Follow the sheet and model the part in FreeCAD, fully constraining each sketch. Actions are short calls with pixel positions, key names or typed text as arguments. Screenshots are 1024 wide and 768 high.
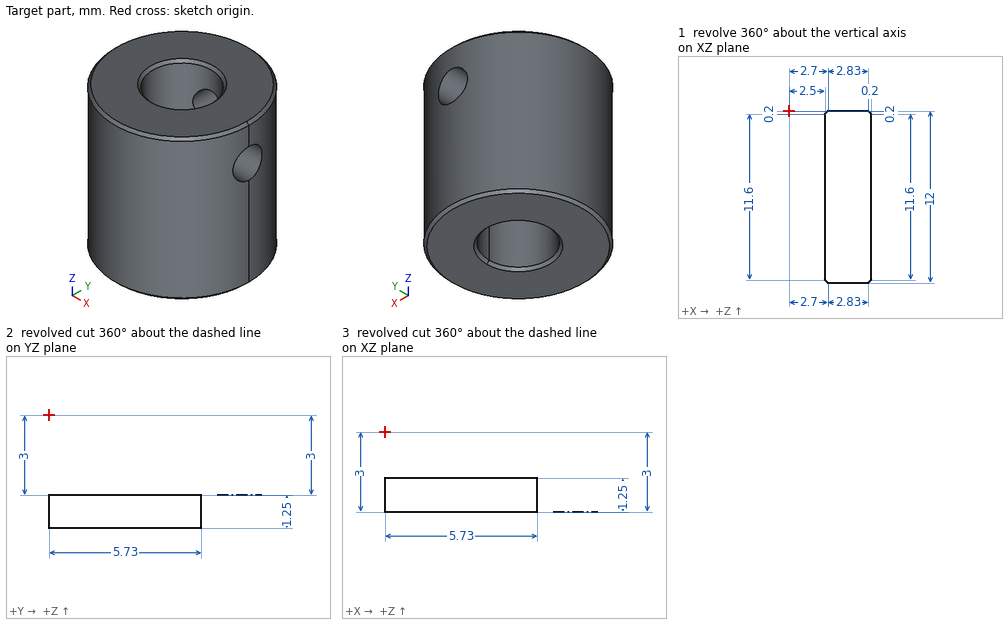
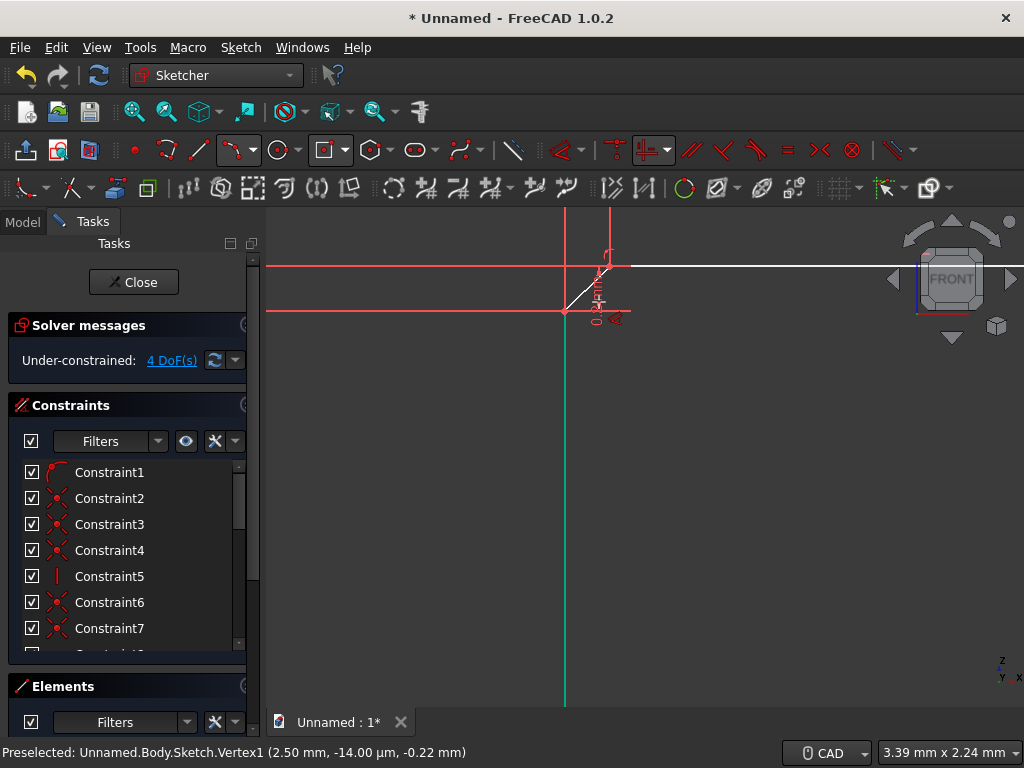
scroll(568, 314, down, 11)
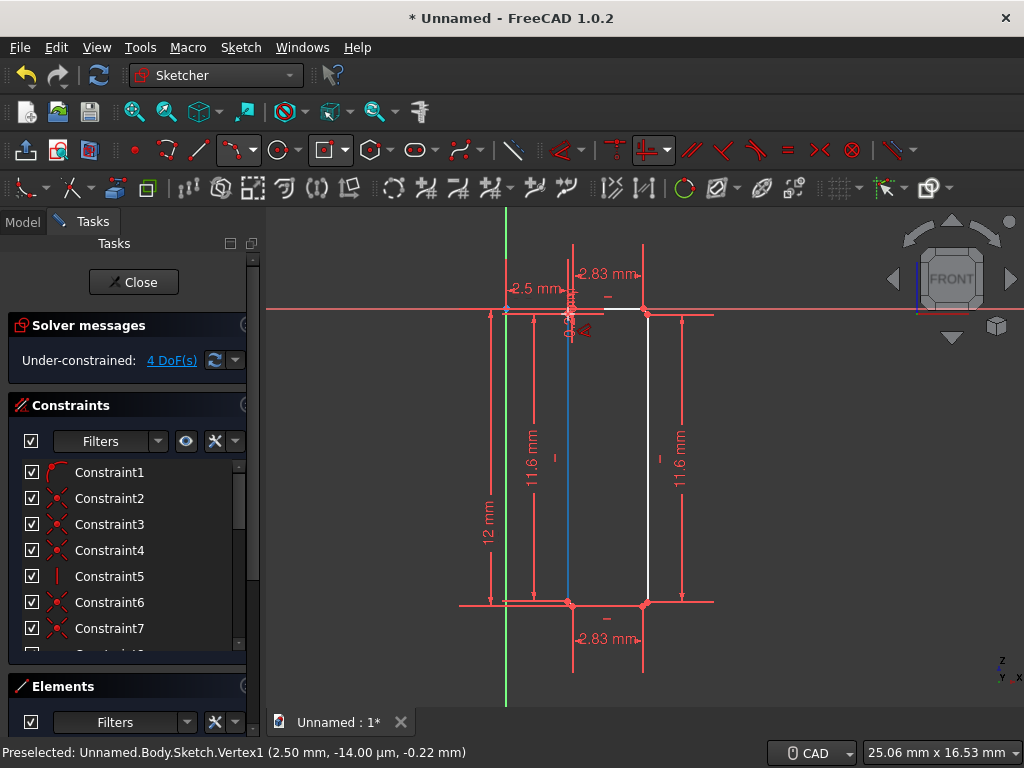
scroll(573, 309, up, 3)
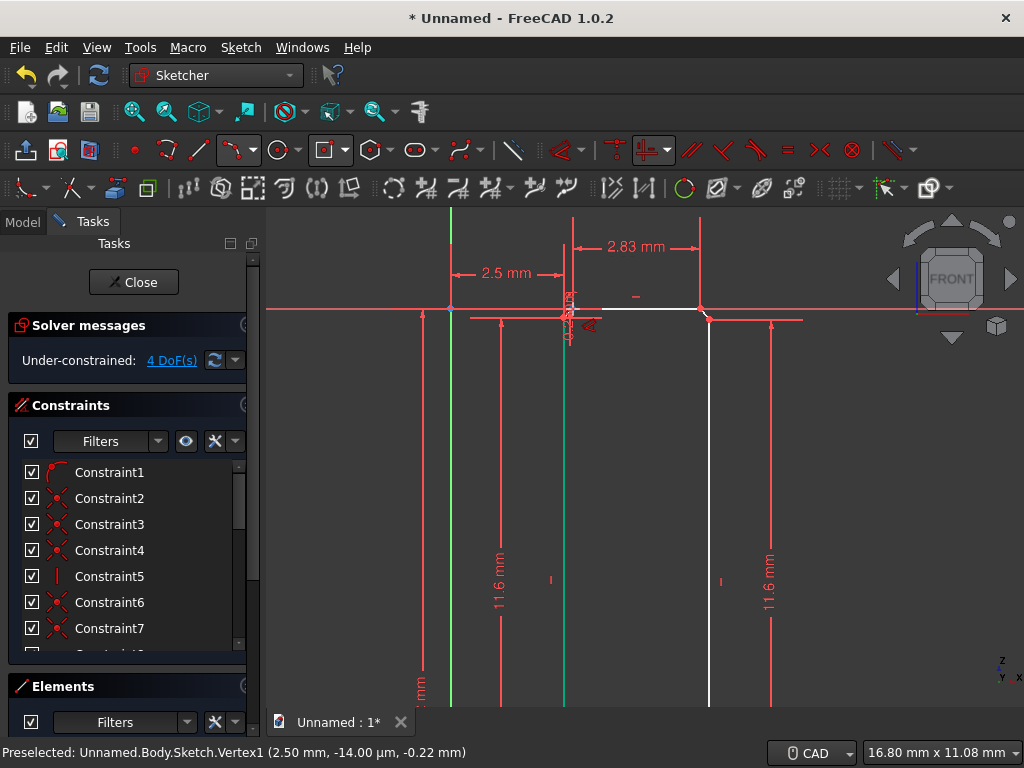
click(573, 309)
click(512, 343)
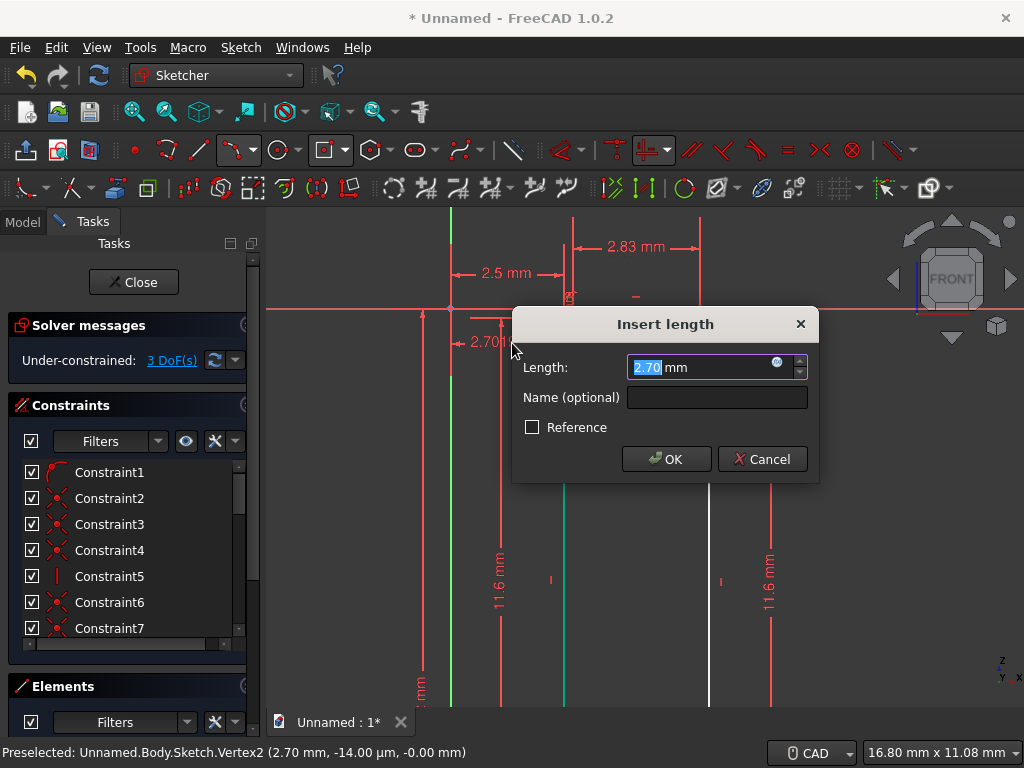
text(2.7)
key(Return)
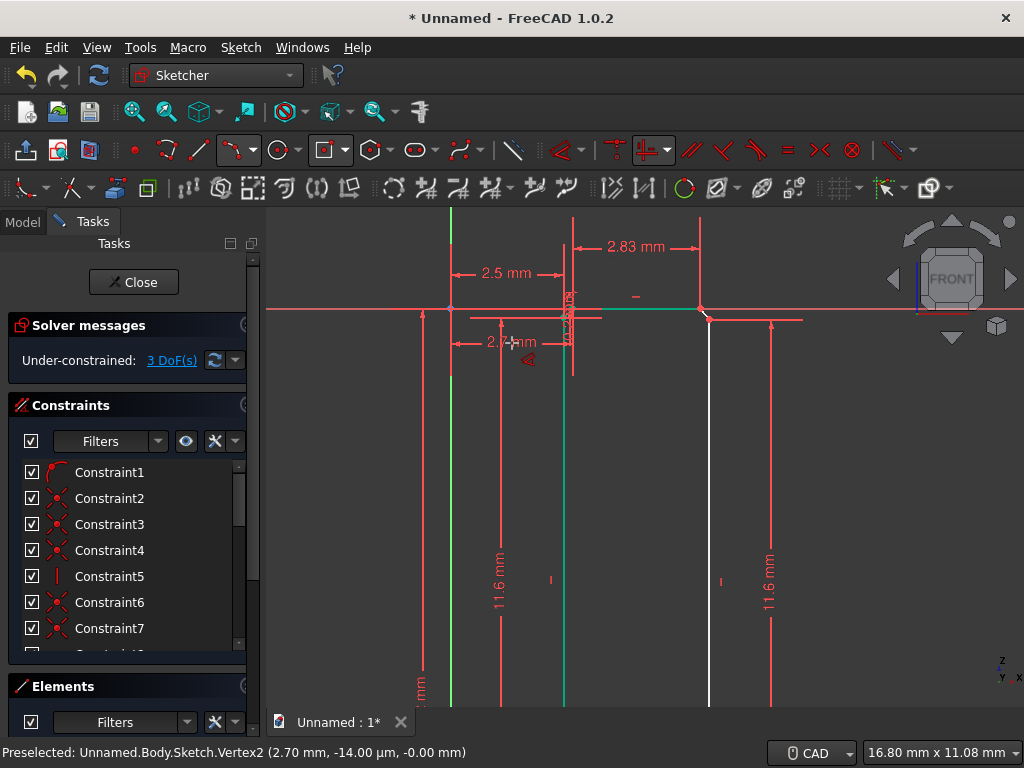
scroll(709, 320, up, 8)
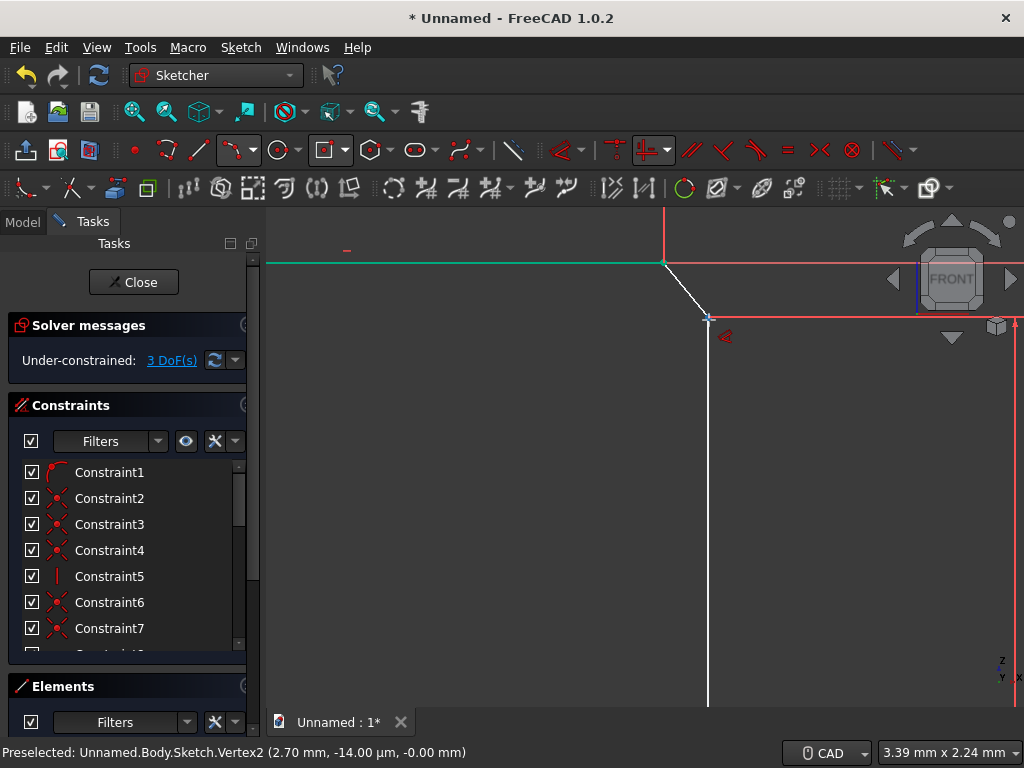
click(708, 317)
click(742, 290)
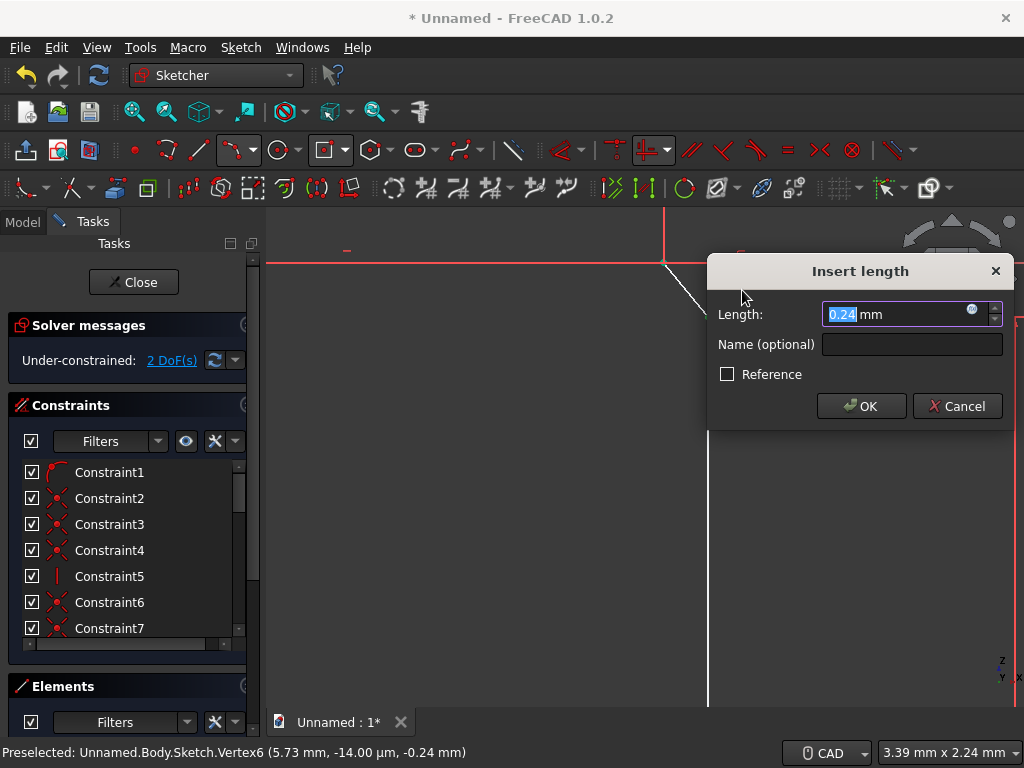
text(0.2)
key(Return)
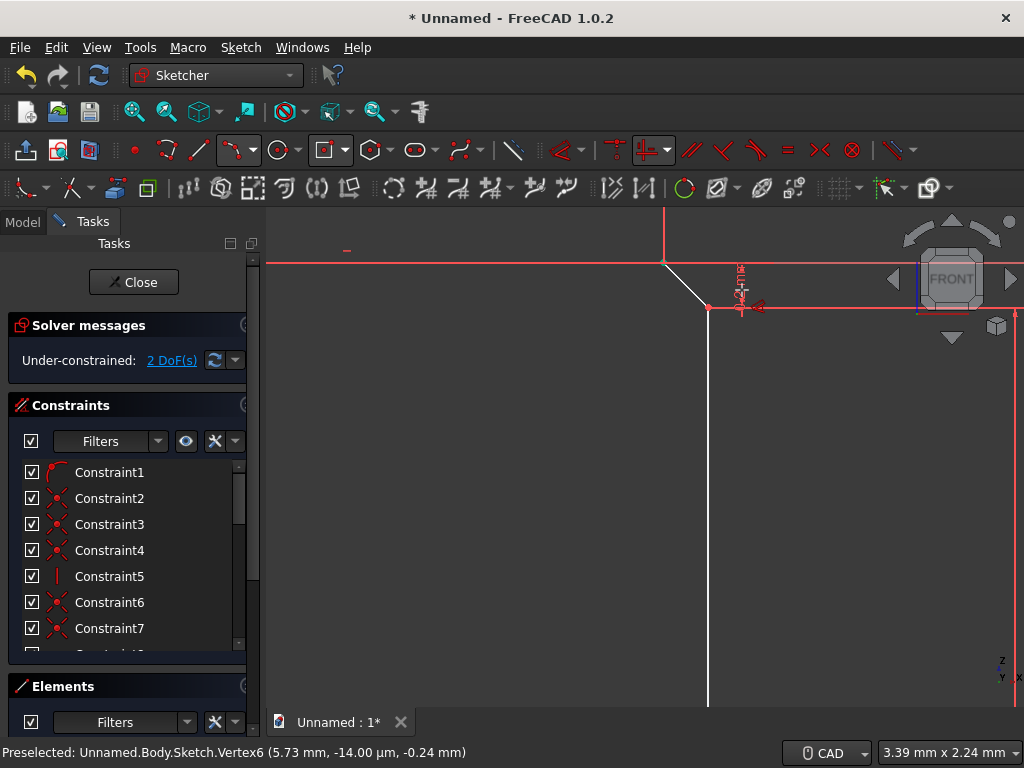
scroll(640, 314, down, 11)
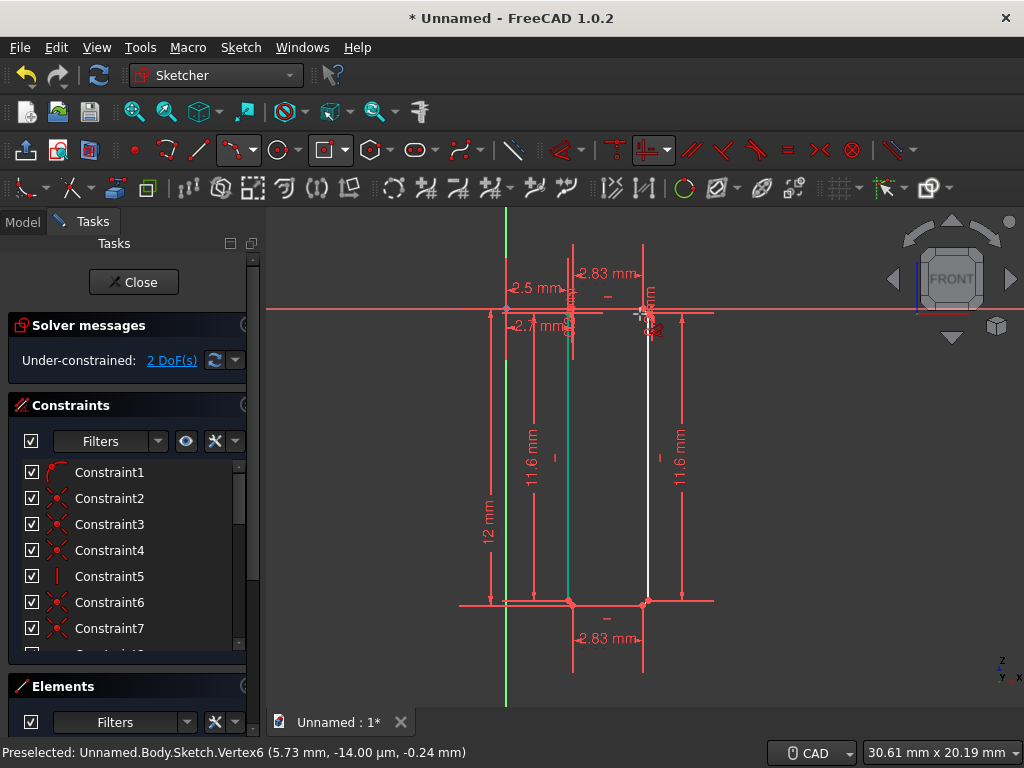
scroll(573, 606, up, 3)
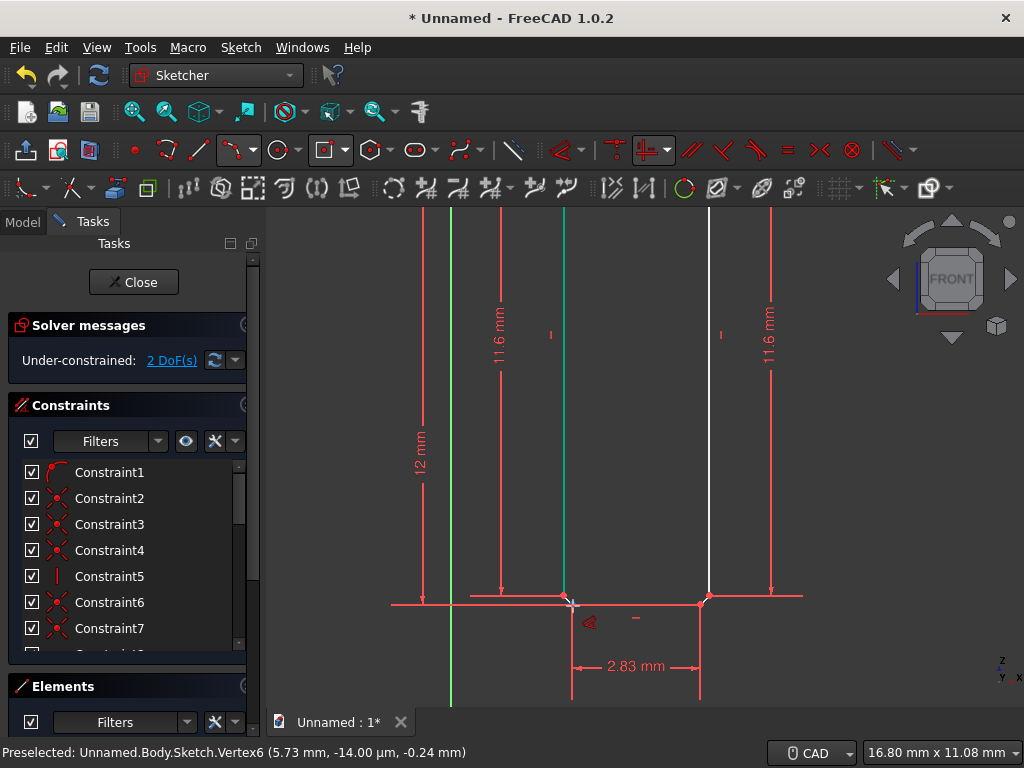
click(572, 605)
click(512, 639)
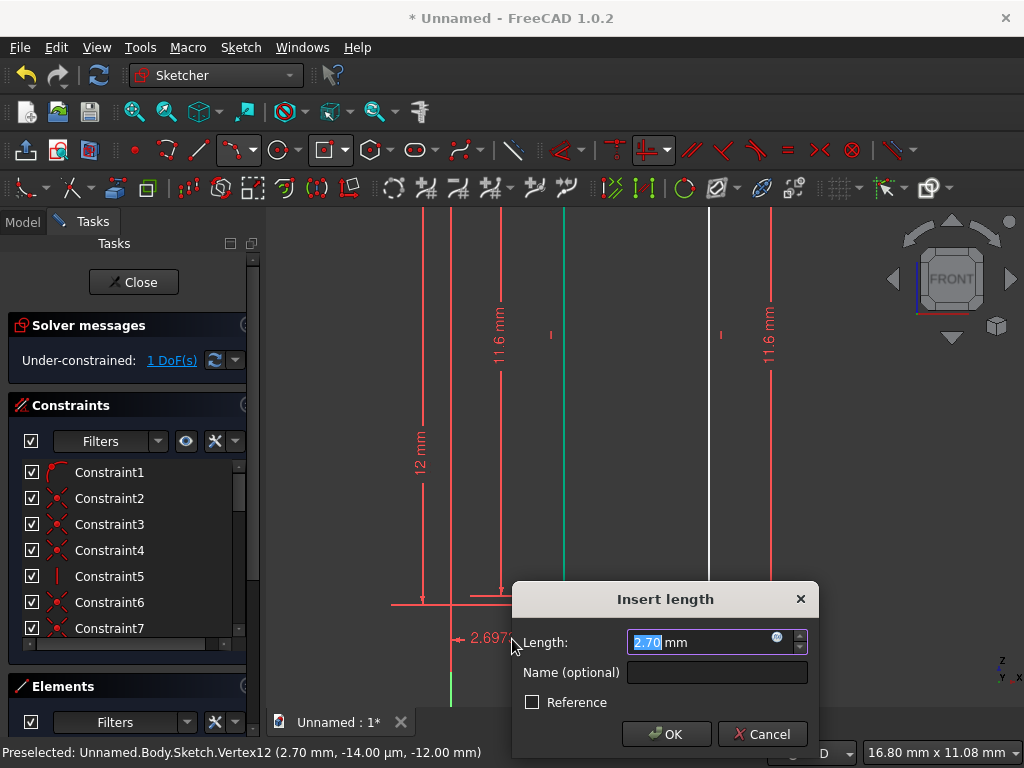
text(2.7)
key(Return)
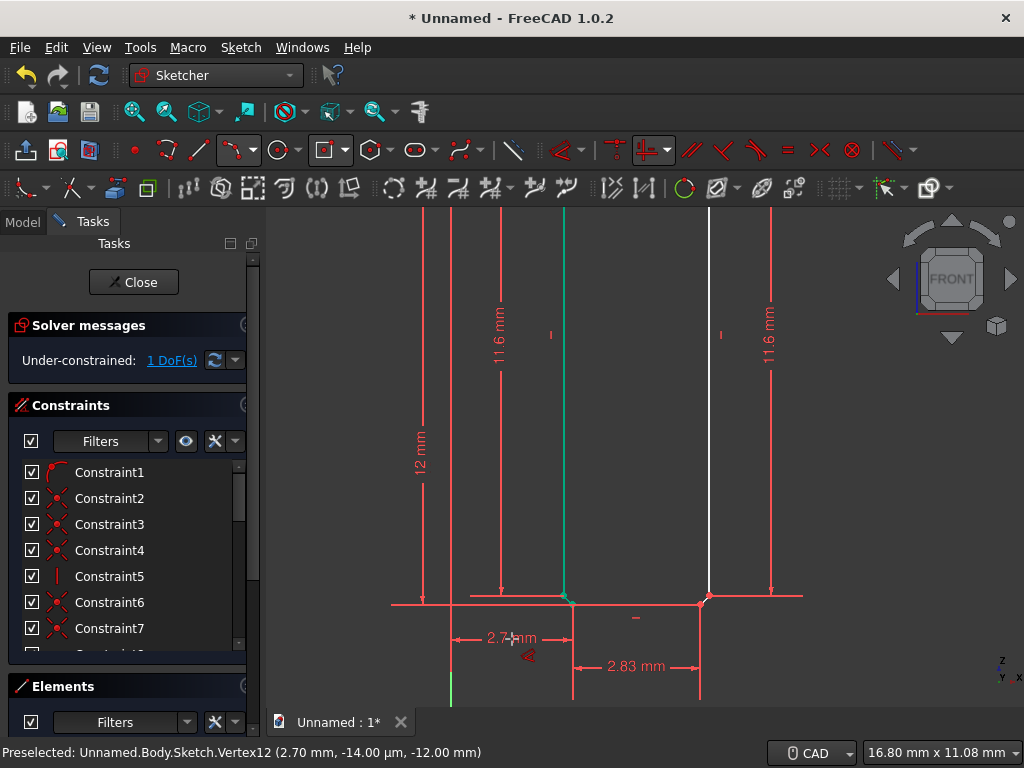
scroll(572, 607, down, 3)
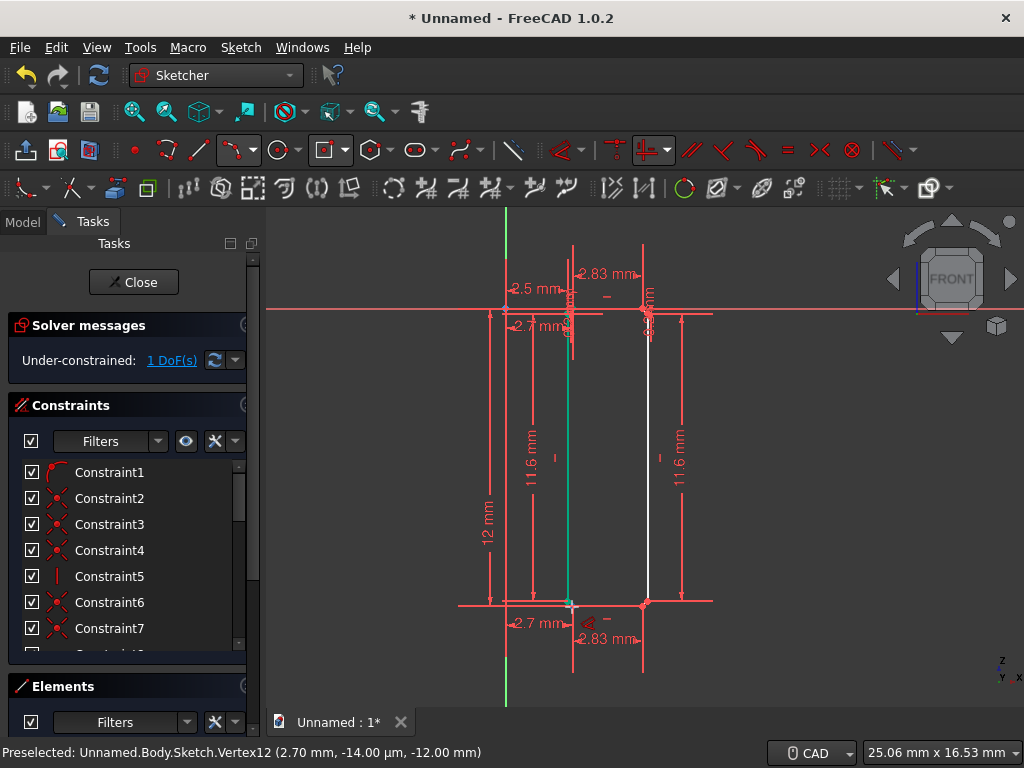
scroll(645, 311, up, 11)